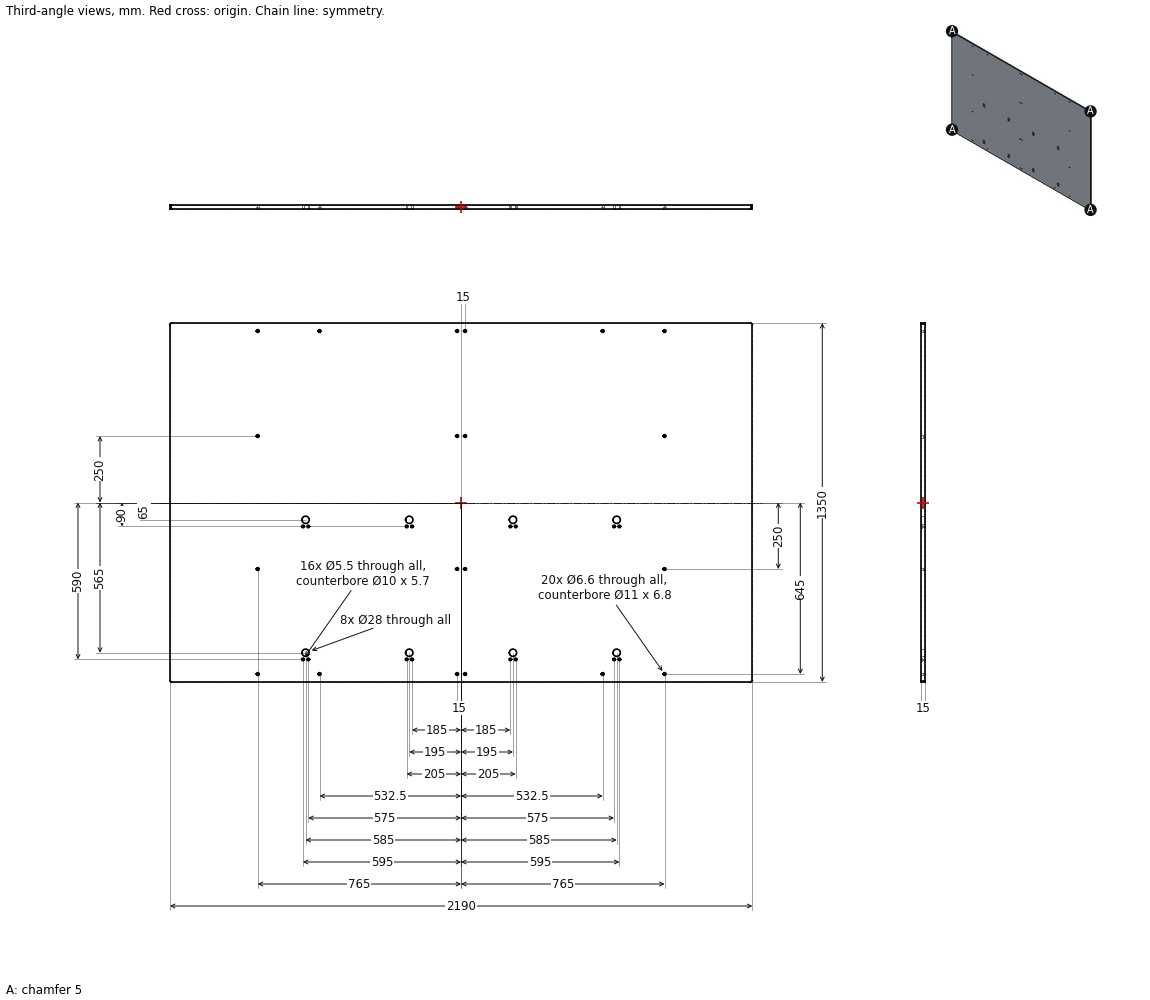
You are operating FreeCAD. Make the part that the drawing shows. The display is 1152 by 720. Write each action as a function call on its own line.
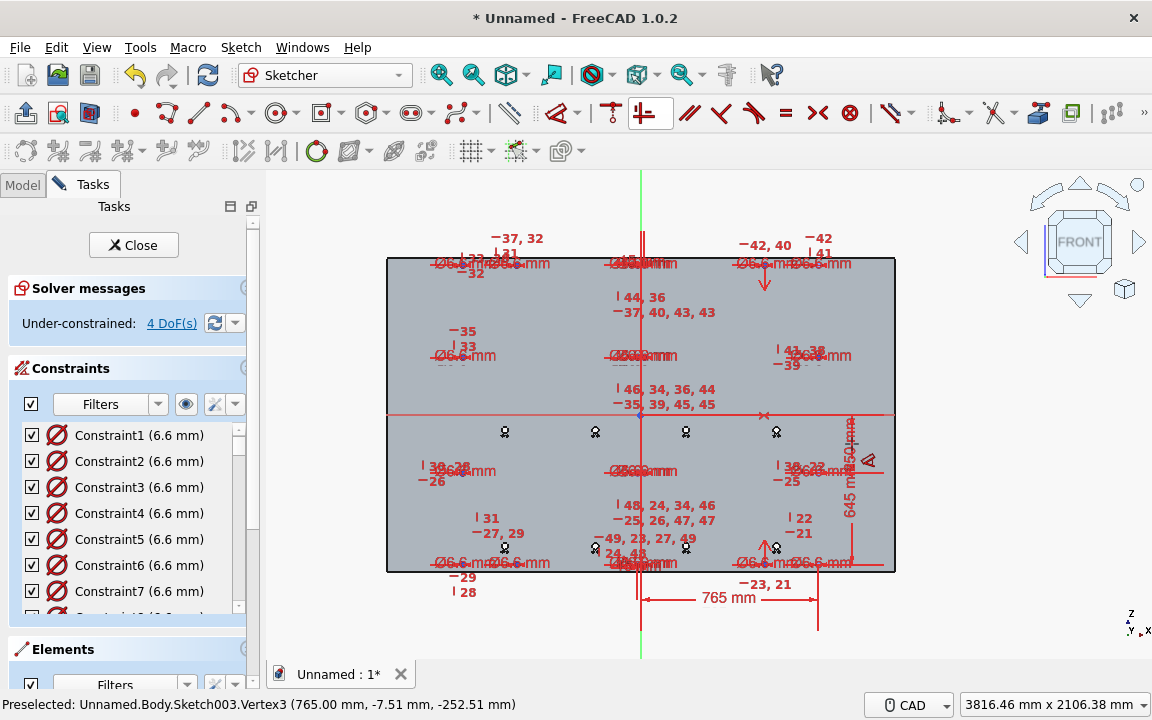
click(463, 473)
click(552, 507)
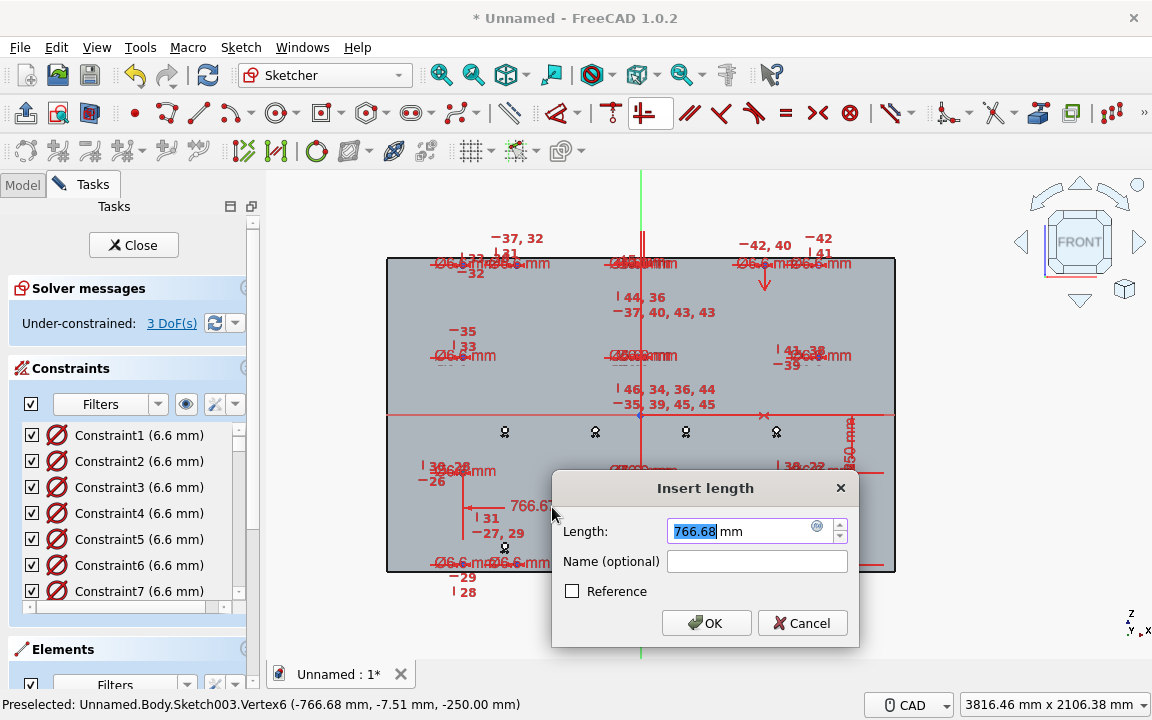
text(765)
key(Return)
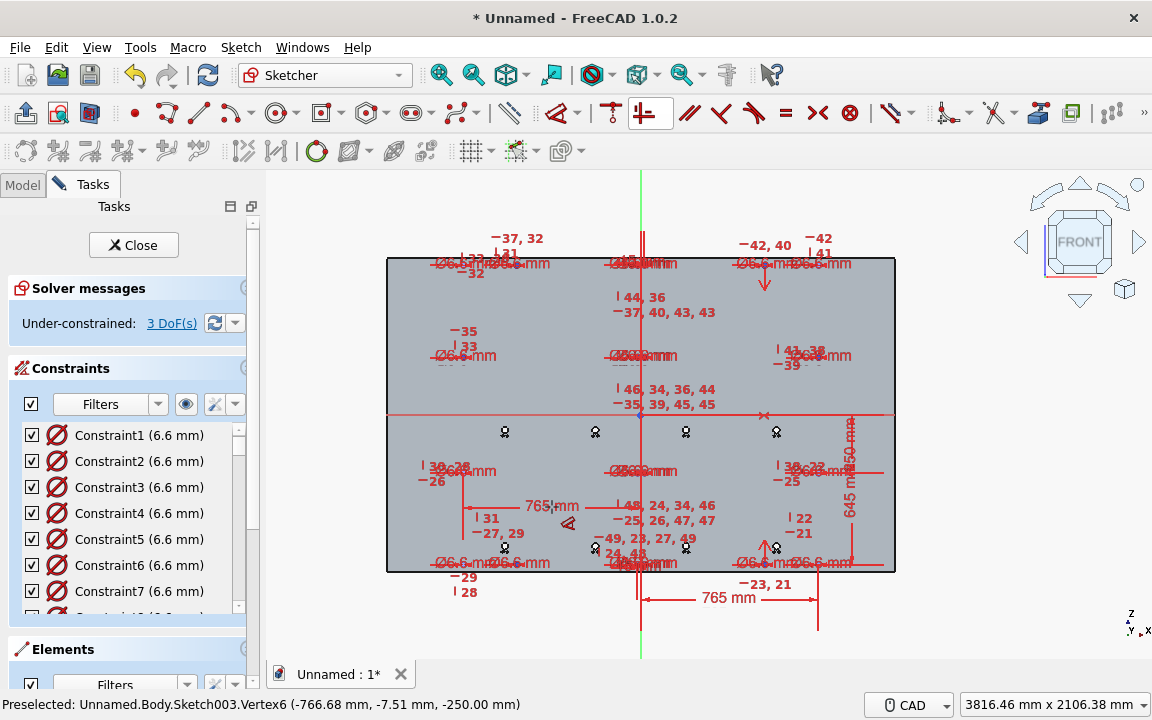
click(463, 358)
click(429, 386)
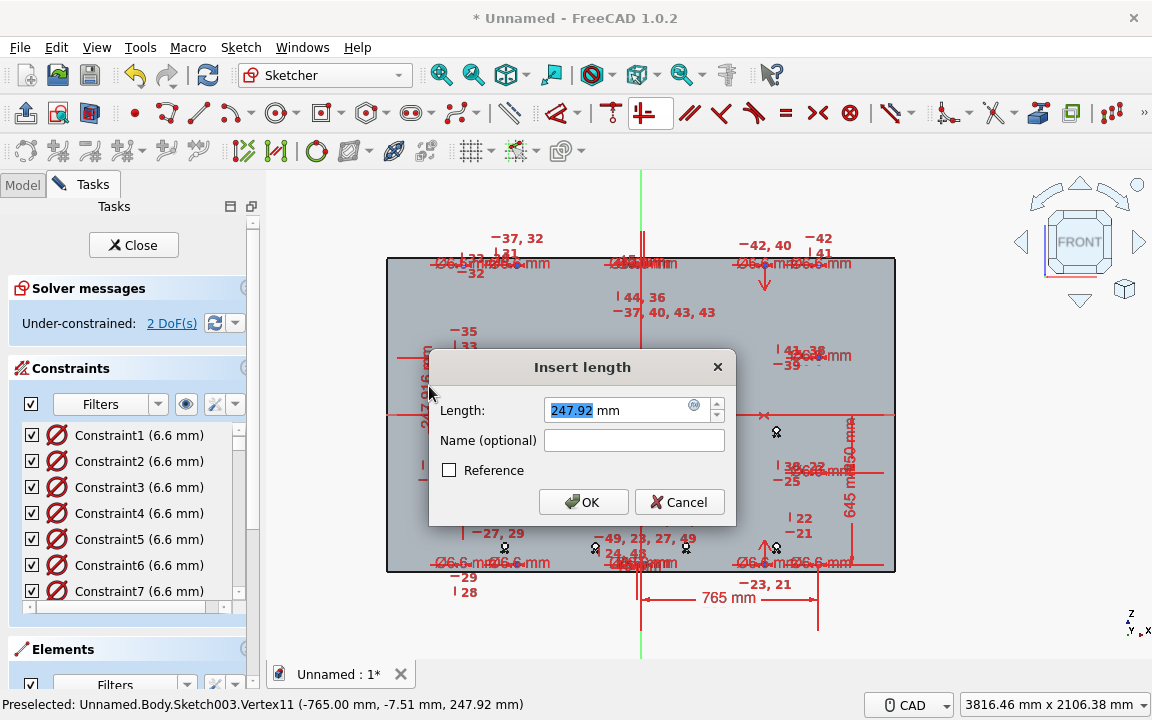
text(250)
key(Return)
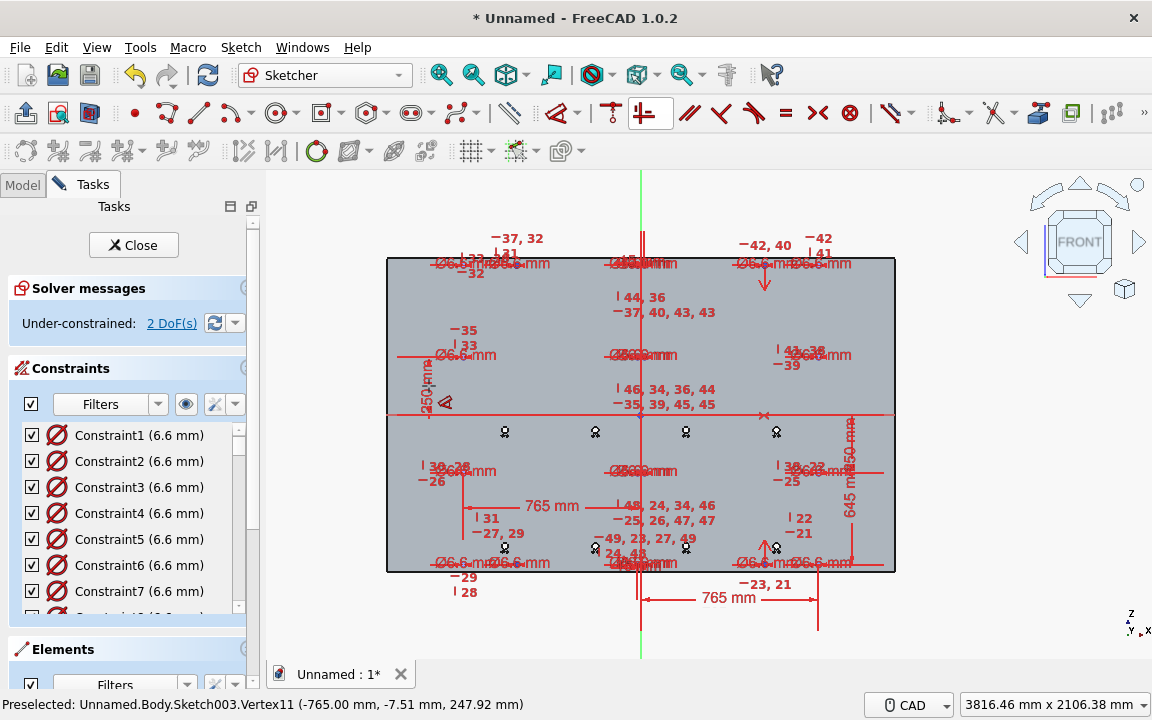
click(765, 565)
click(659, 599)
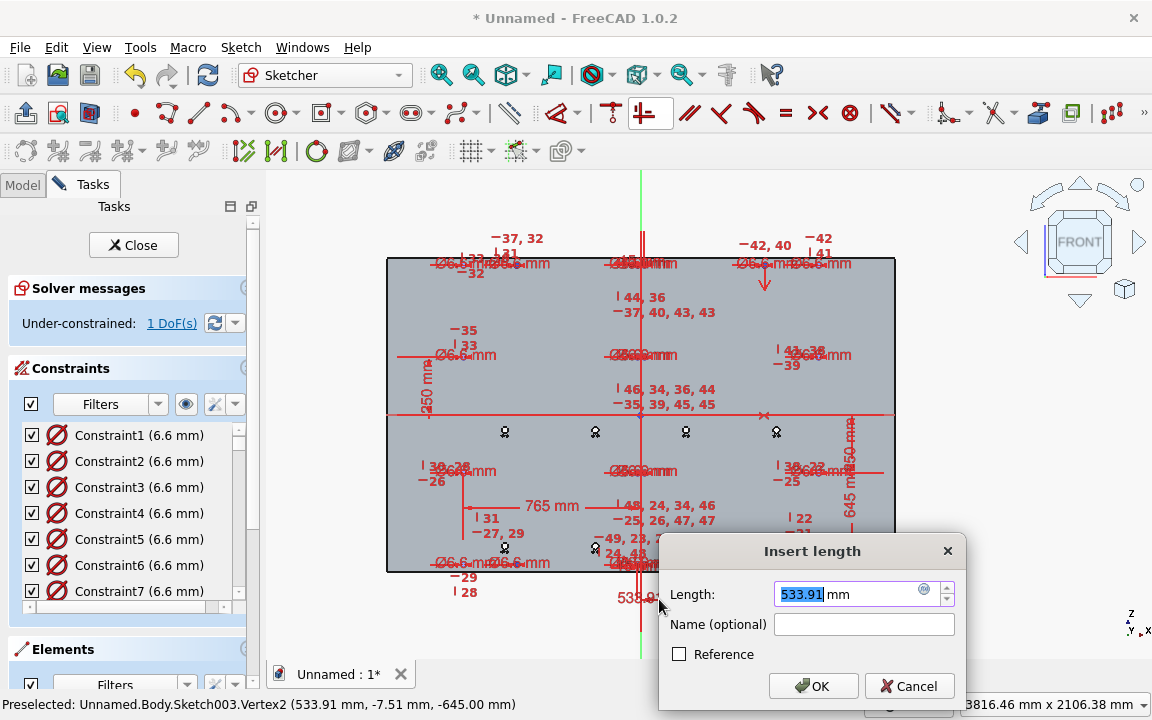
text(532.5)
key(Return)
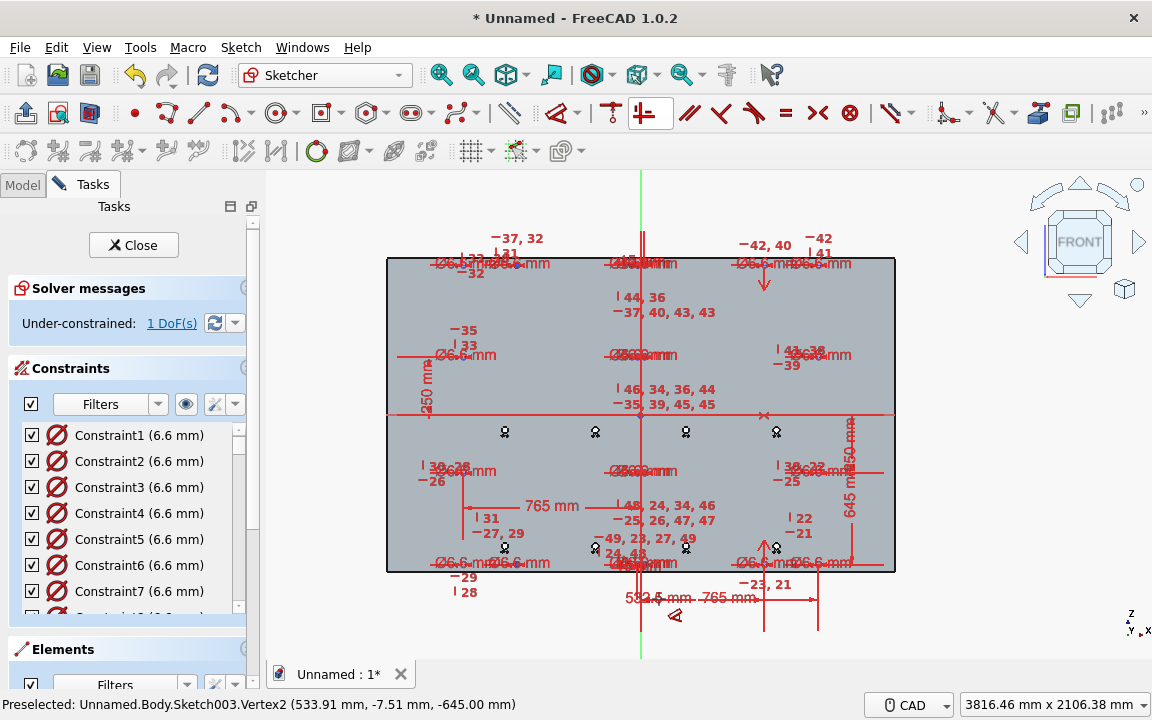
click(517, 565)
click(579, 599)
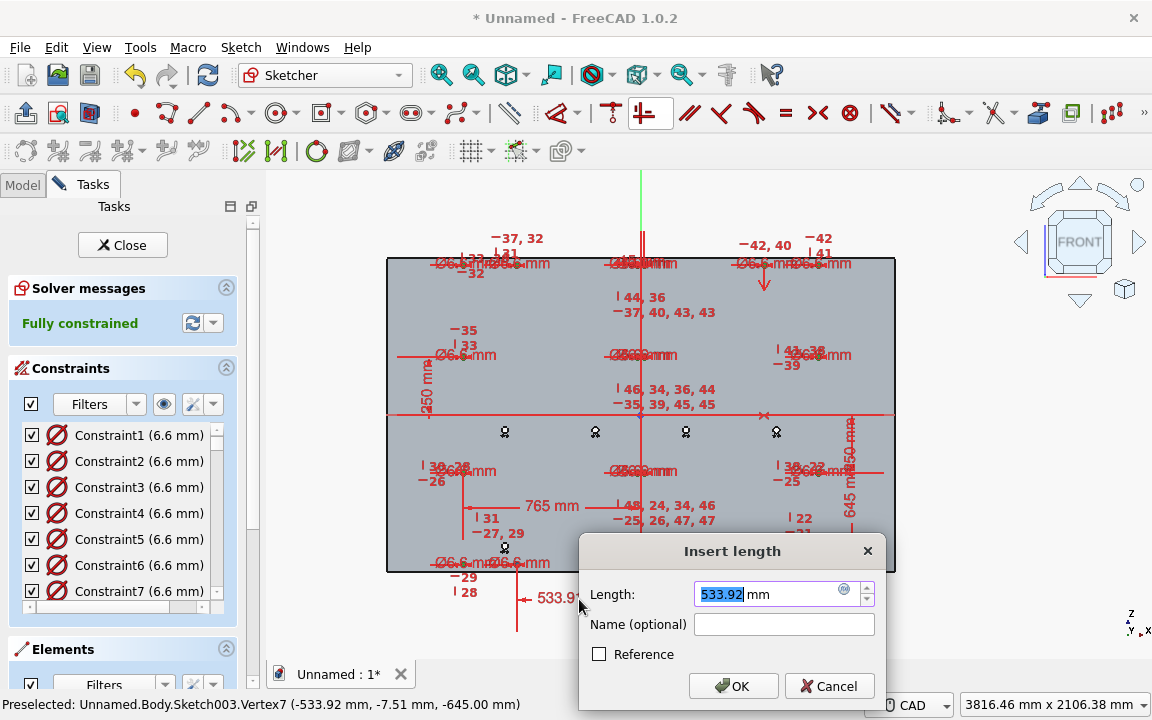
text(532.5)
key(Return)
key(Escape)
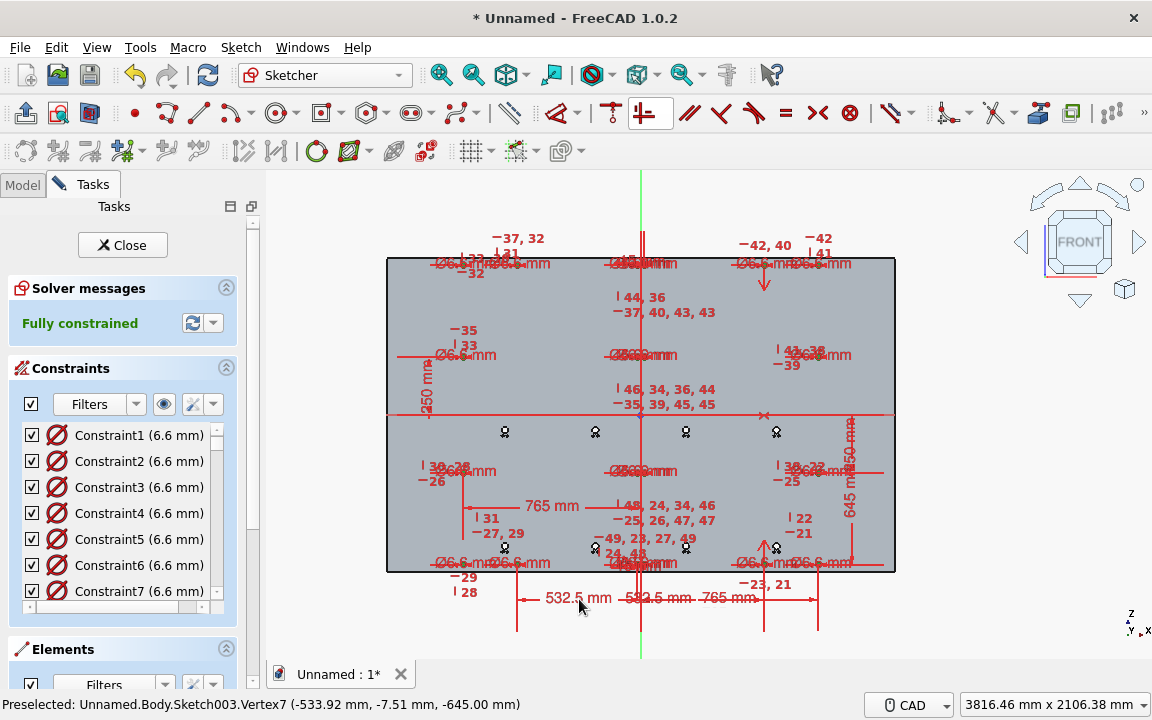
click(123, 245)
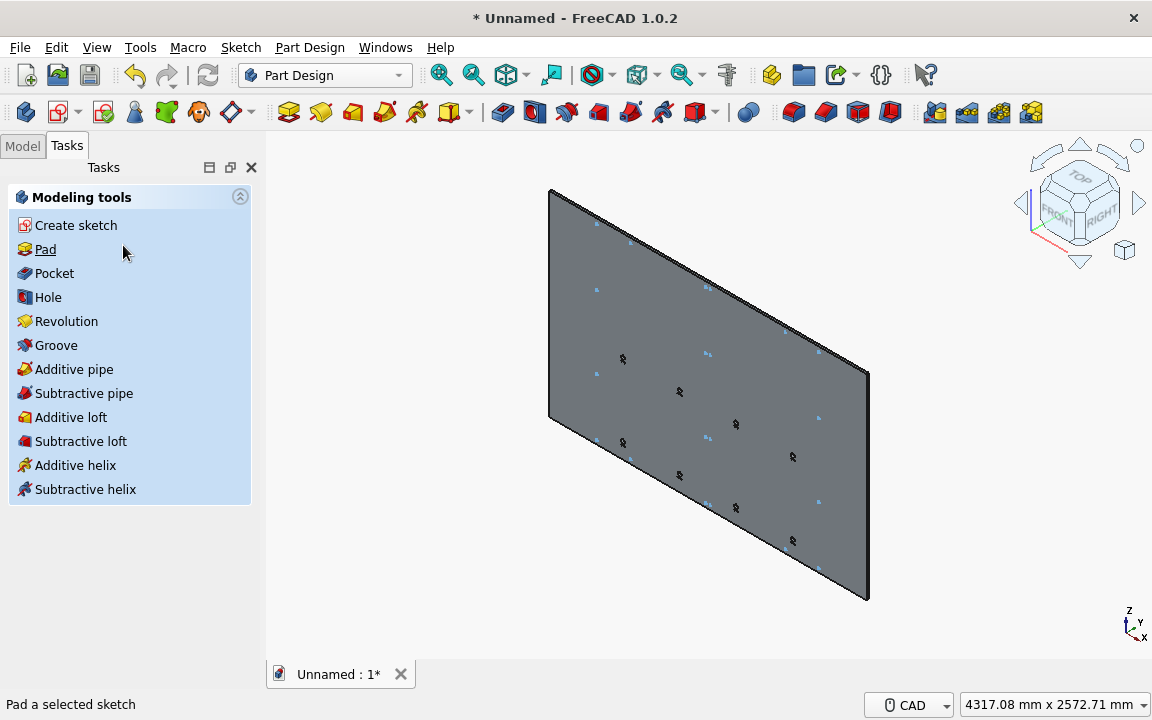
click(536, 112)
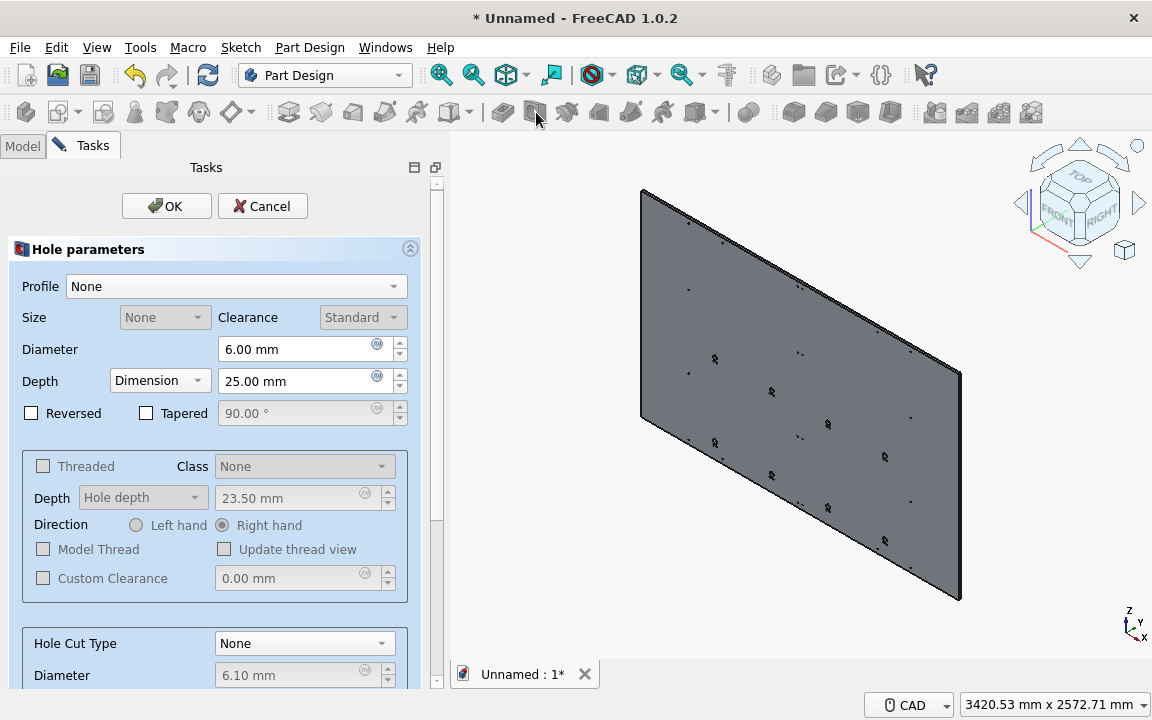
triple_click(305, 349)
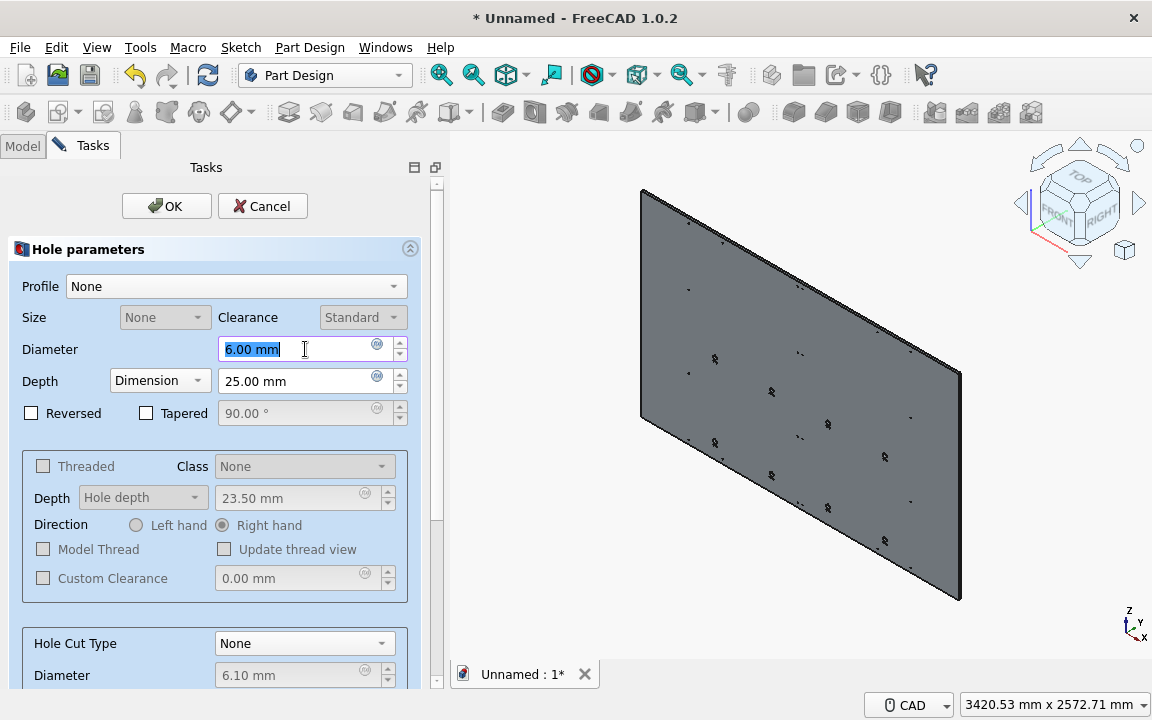
text(6.6)
key(Tab)